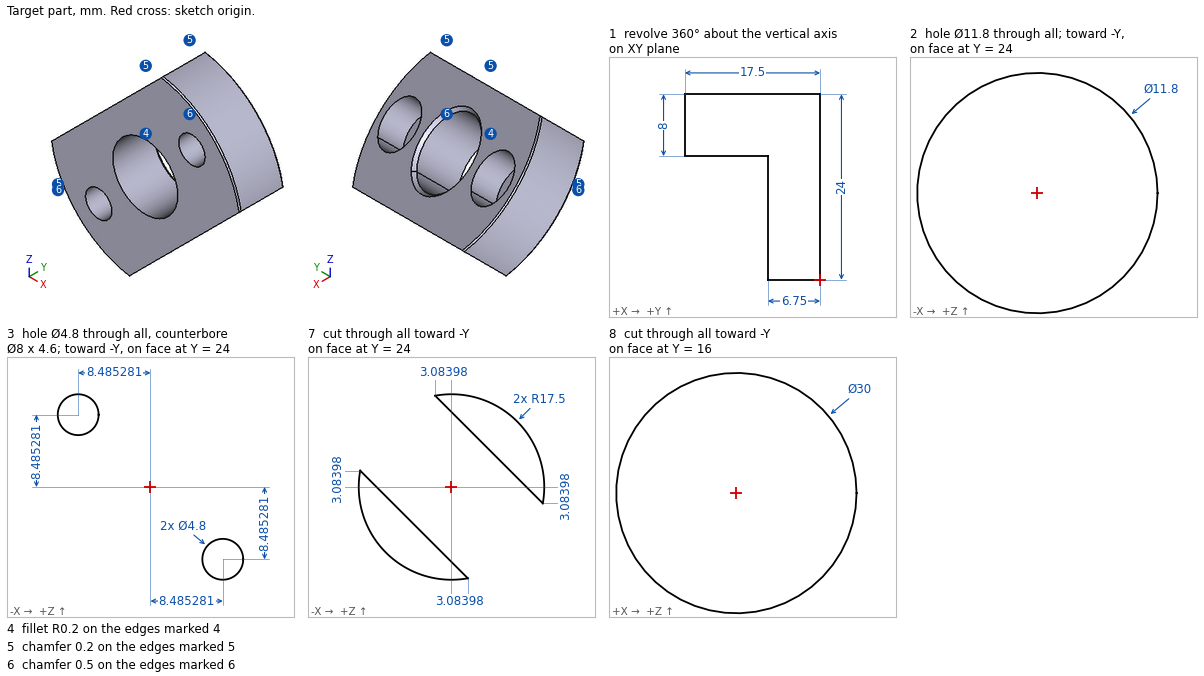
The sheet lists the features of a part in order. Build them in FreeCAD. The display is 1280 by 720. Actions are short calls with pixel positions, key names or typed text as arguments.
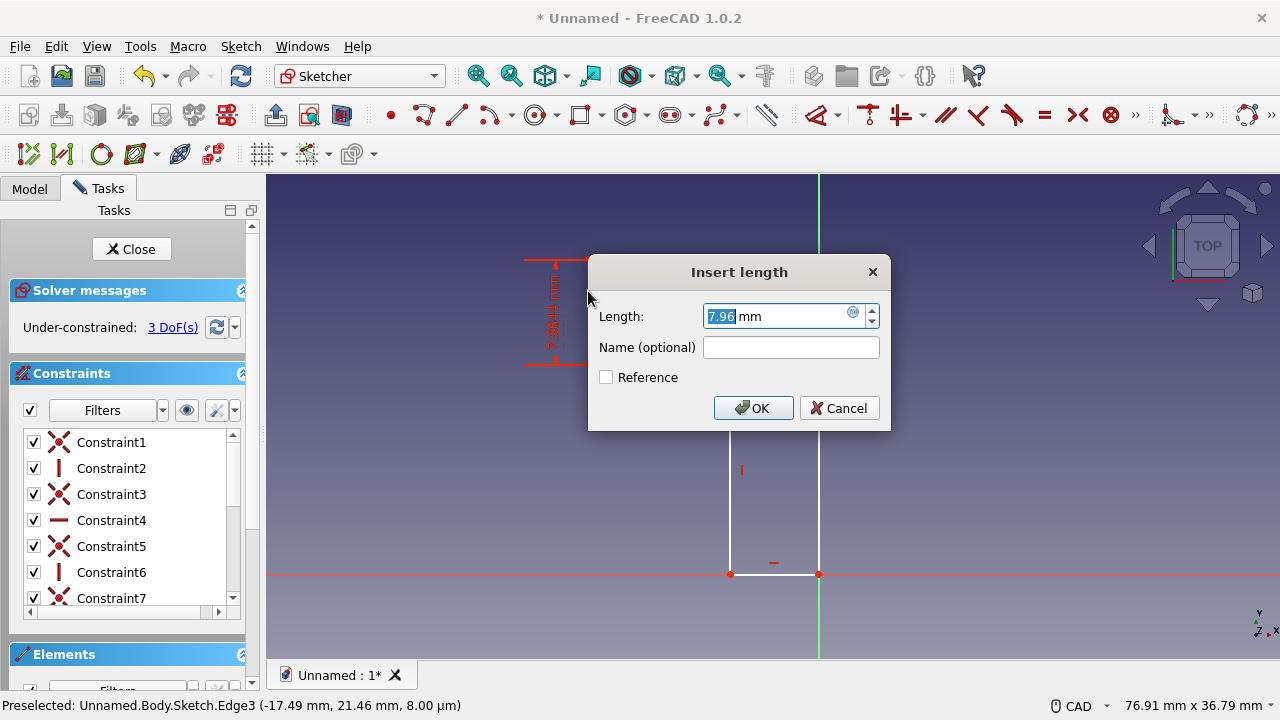
text(8)
key(Return)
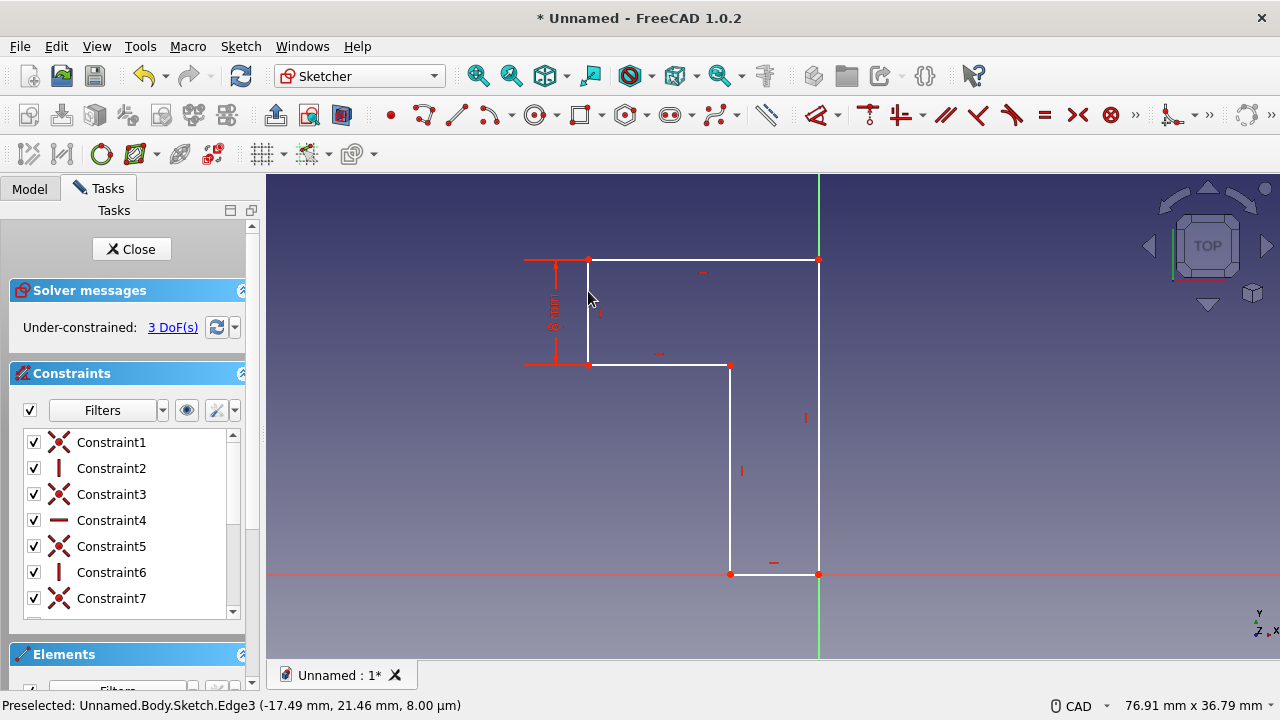
click(819, 480)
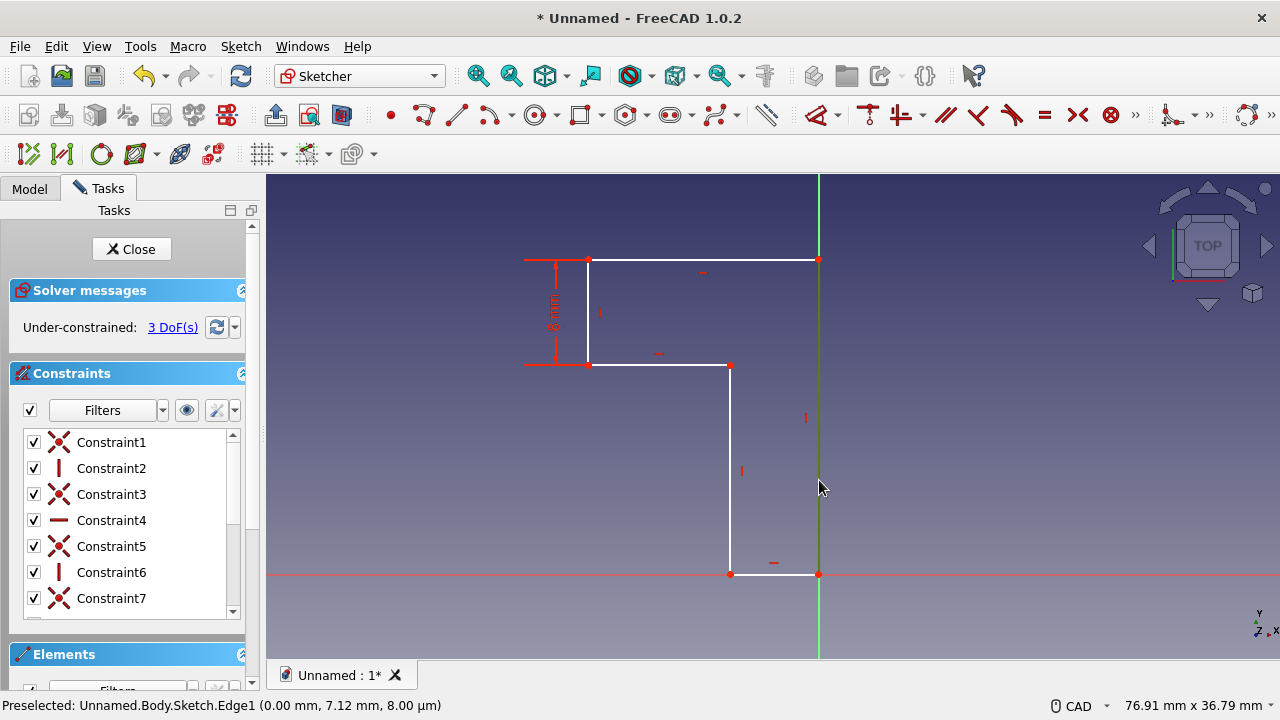
key(i)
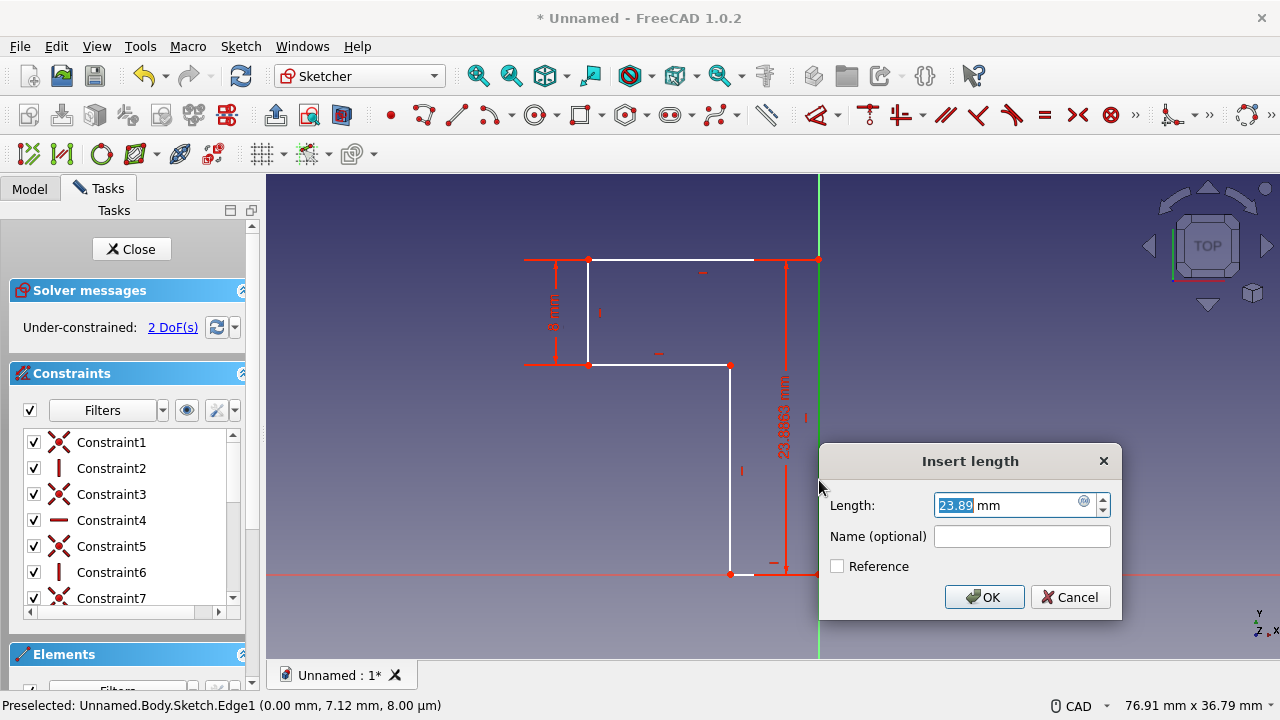
text(24)
key(Return)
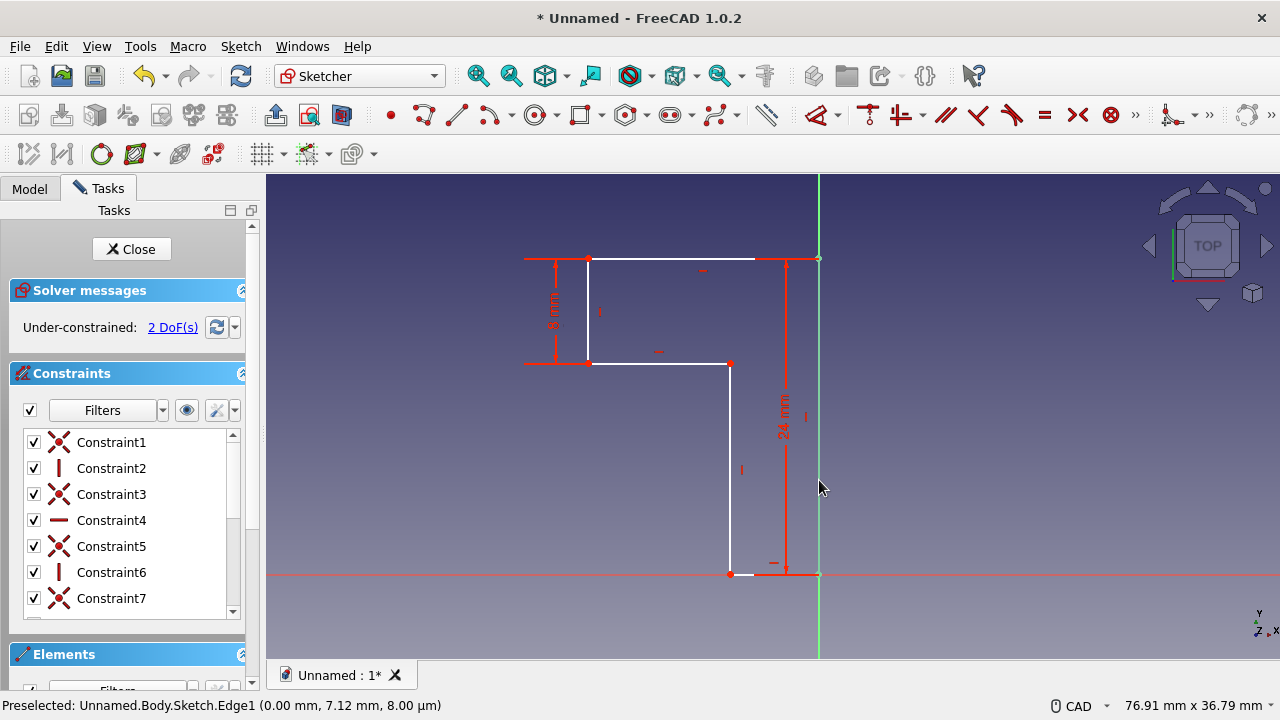
click(749, 259)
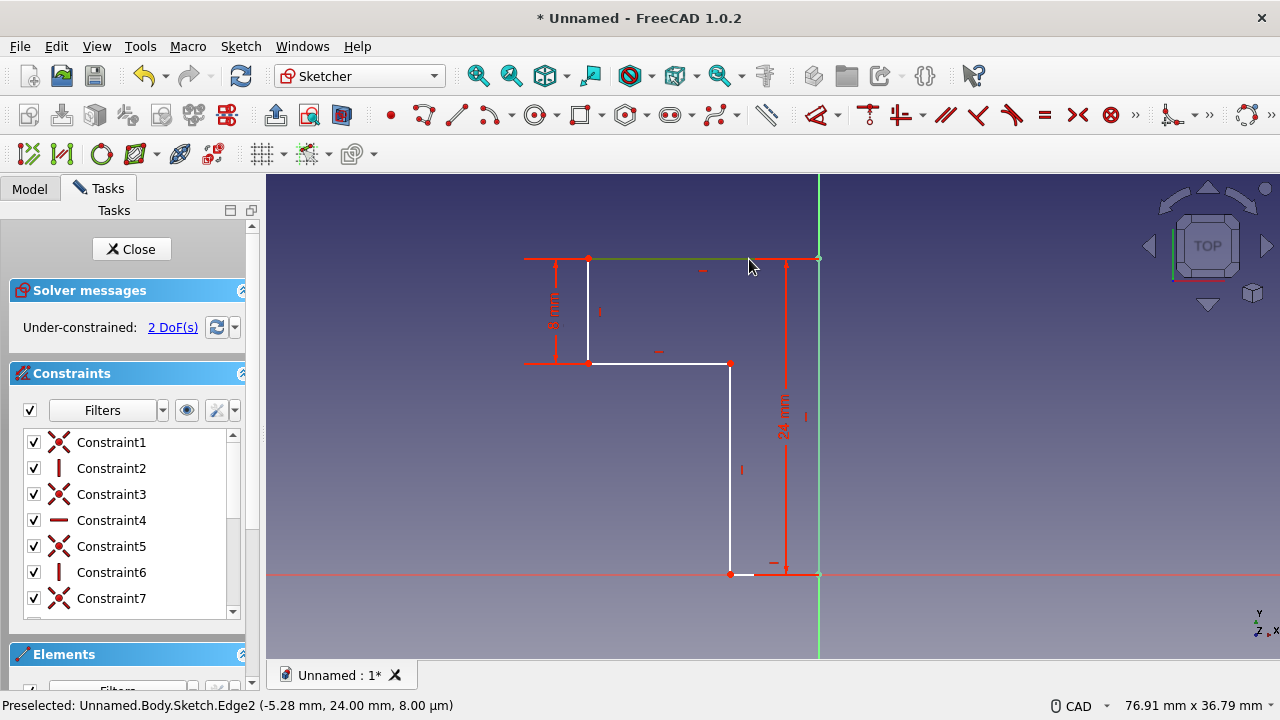
key(l)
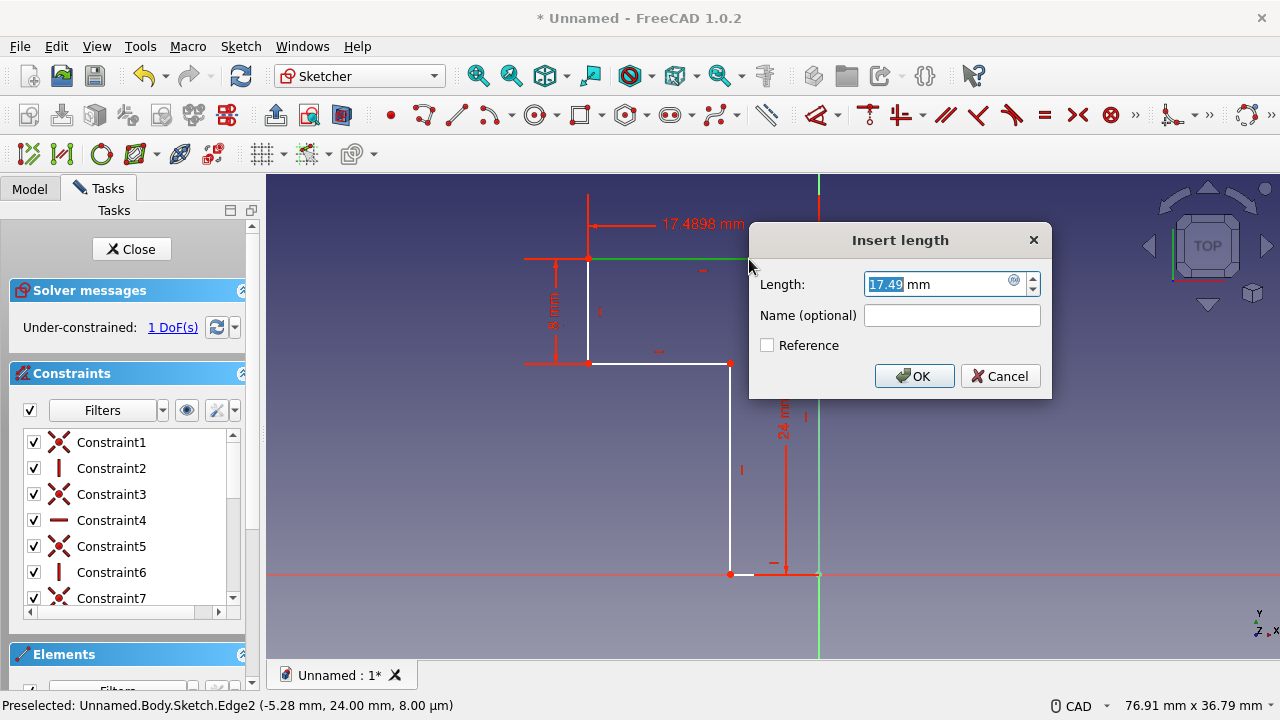
text(17.5)
key(Return)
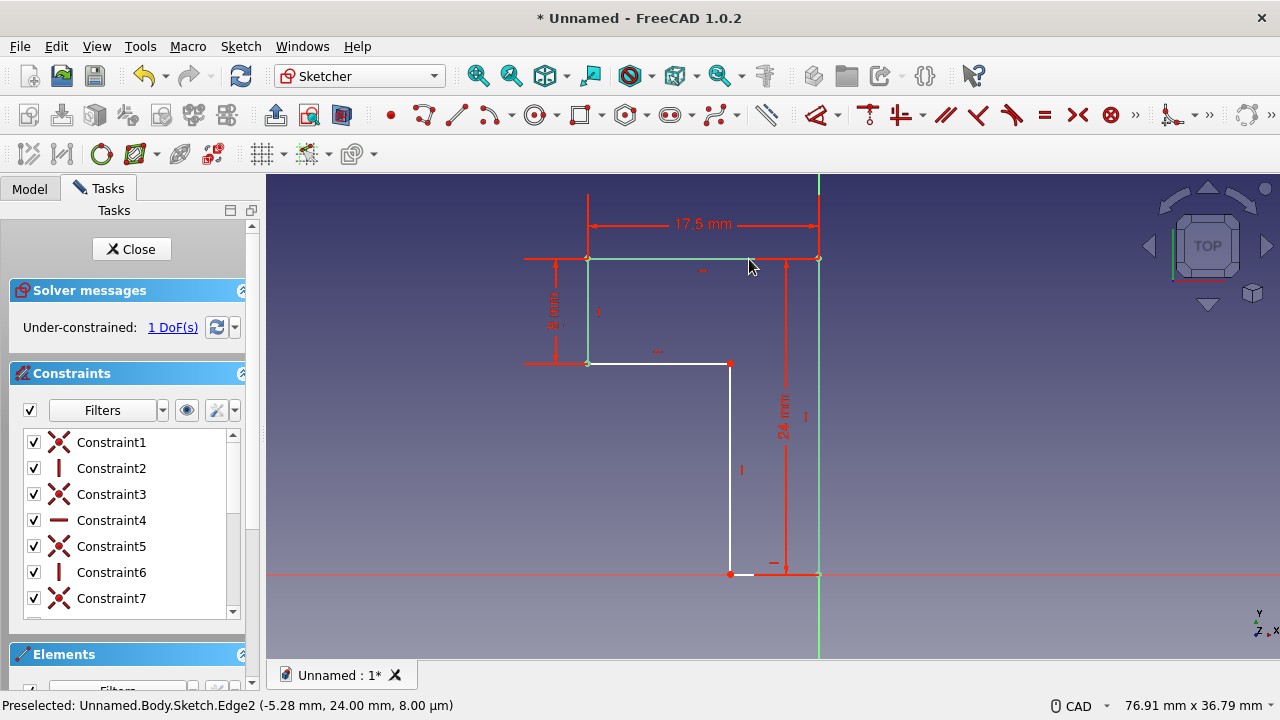
click(757, 575)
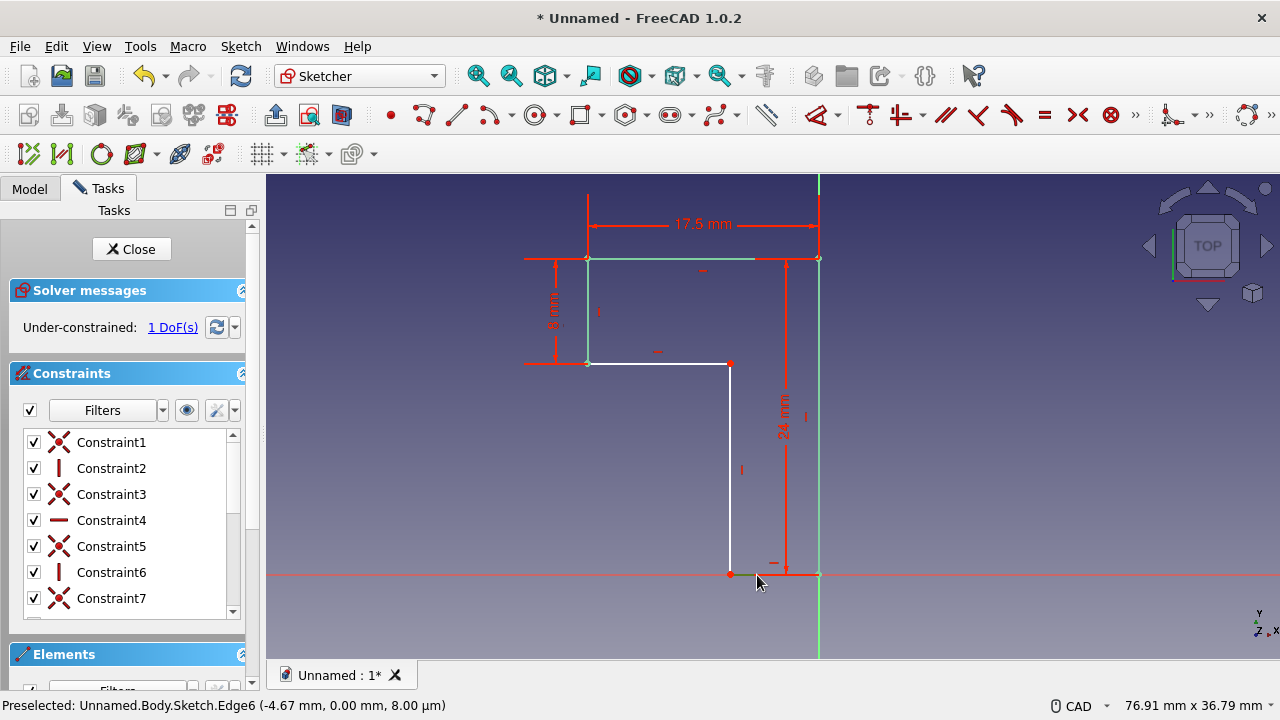
click(838, 116)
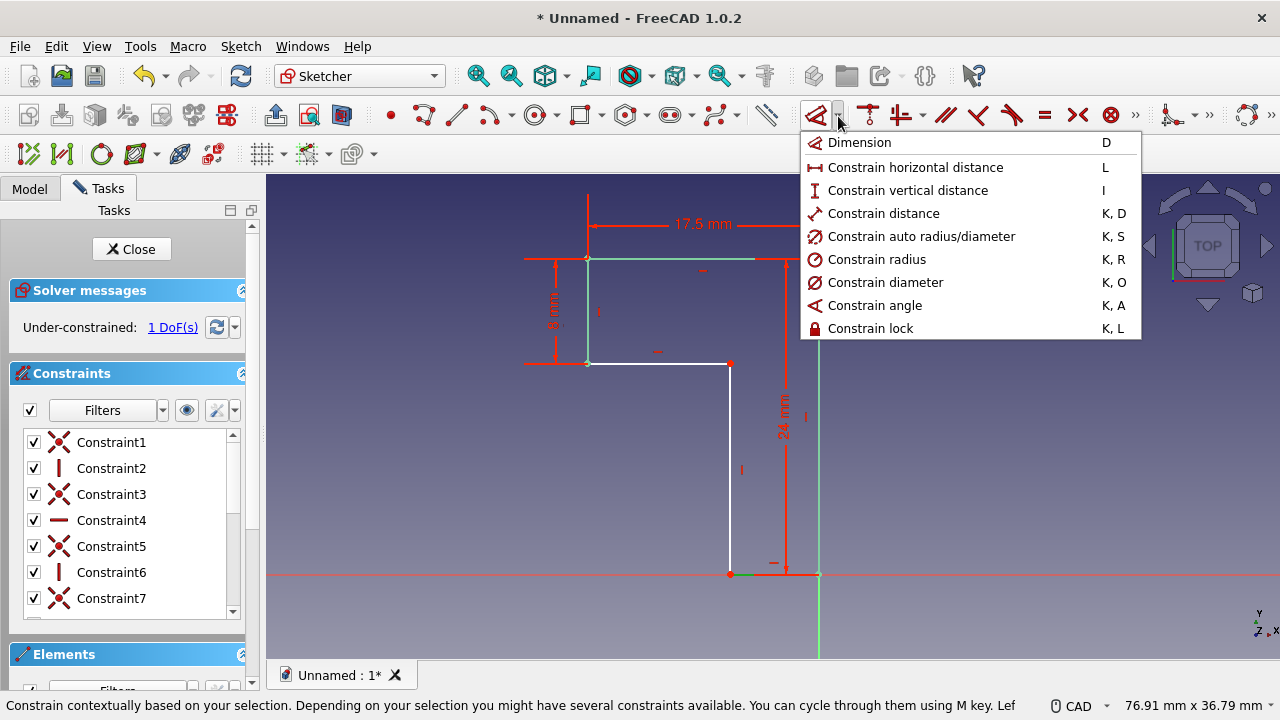
click(971, 168)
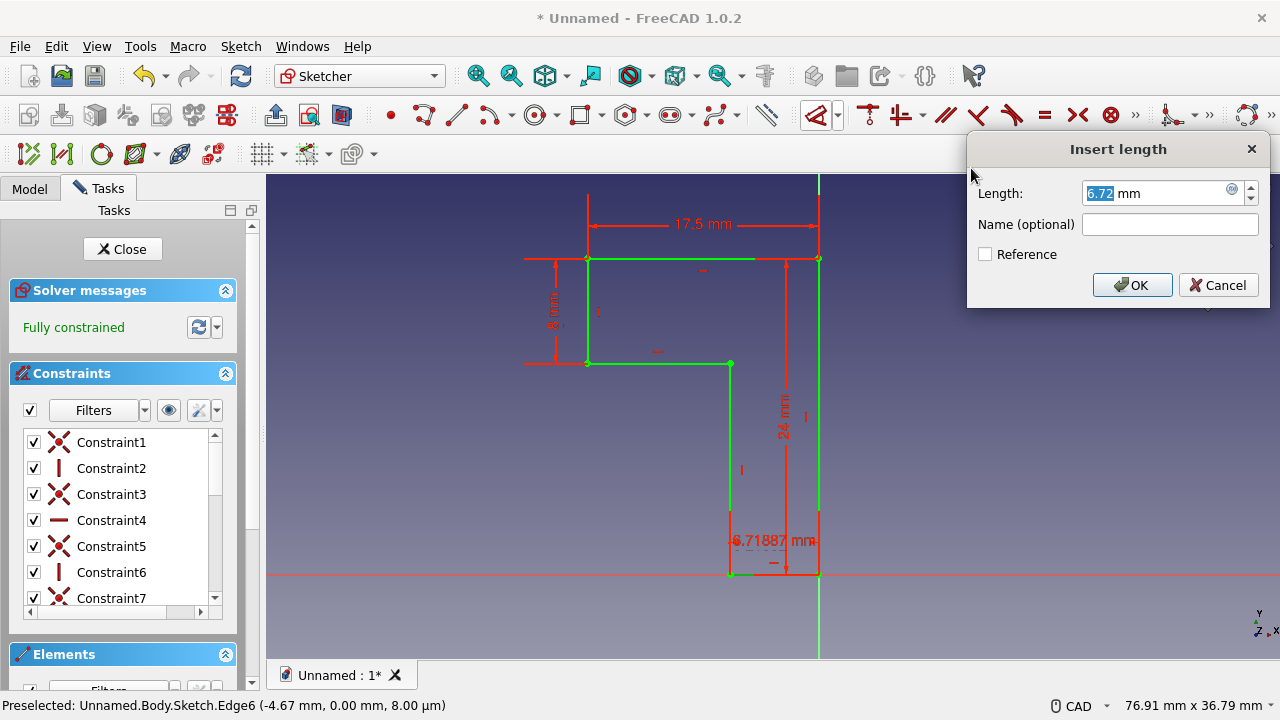
text(6.75)
key(Return)